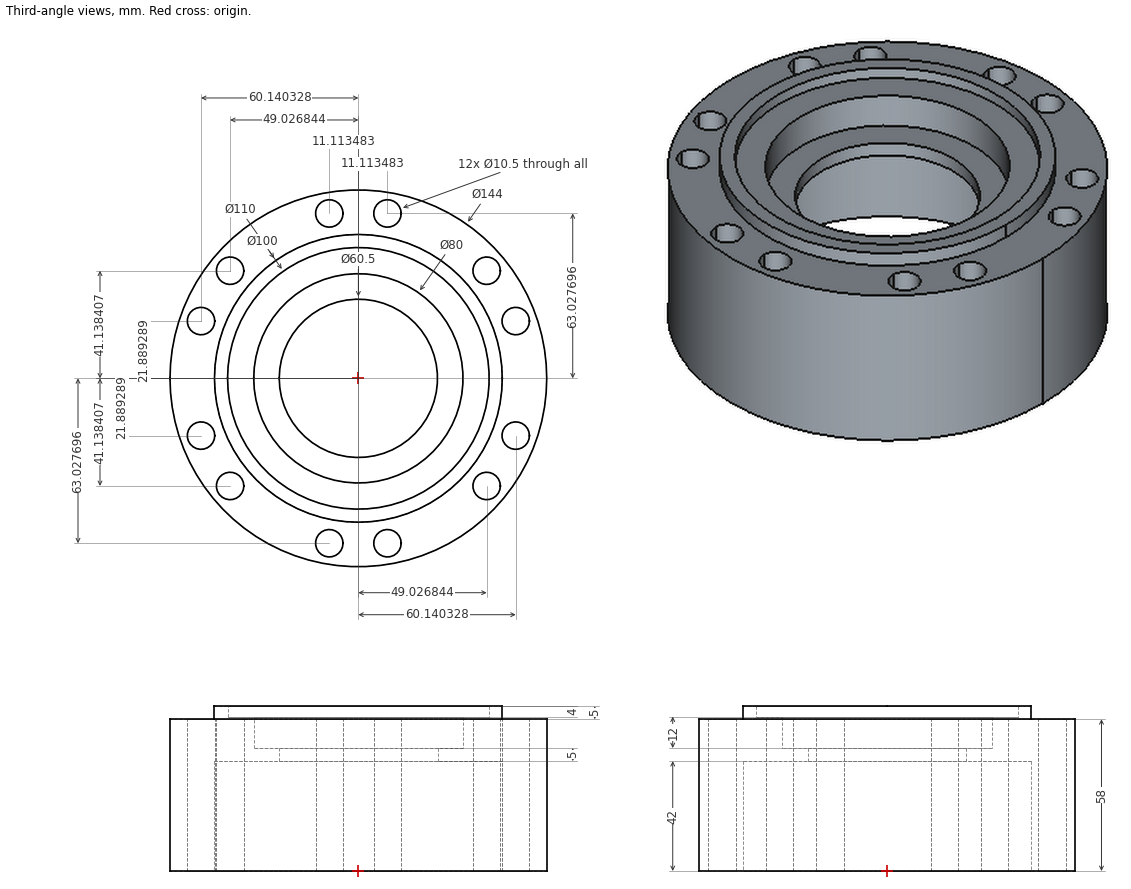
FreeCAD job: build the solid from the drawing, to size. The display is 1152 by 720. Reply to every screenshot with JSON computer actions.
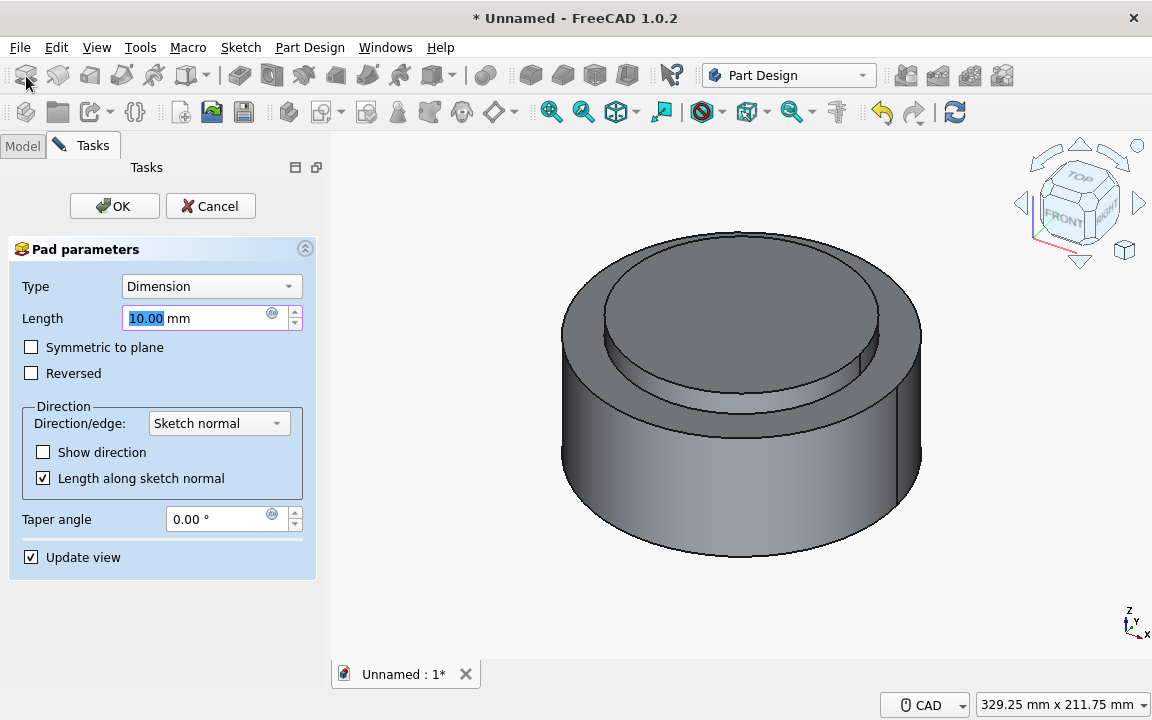
{"action": "type", "text": "5"}
{"action": "key", "text": "Tab"}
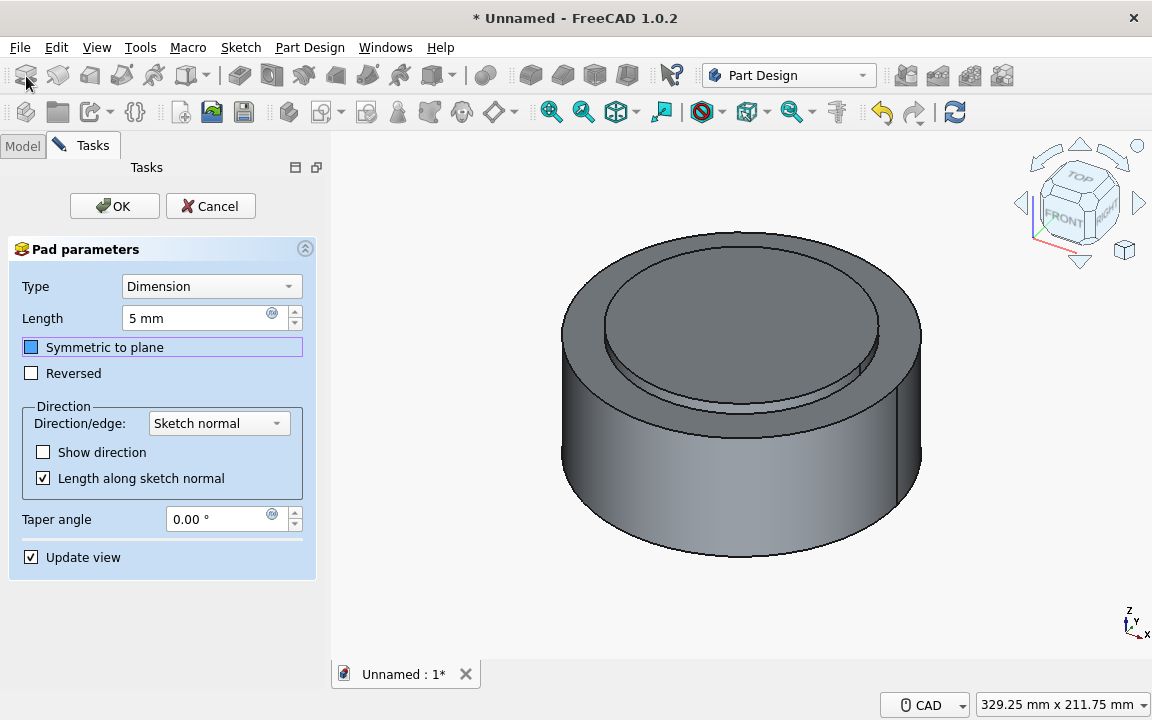
{"action": "left_click", "coordinate": [115, 206]}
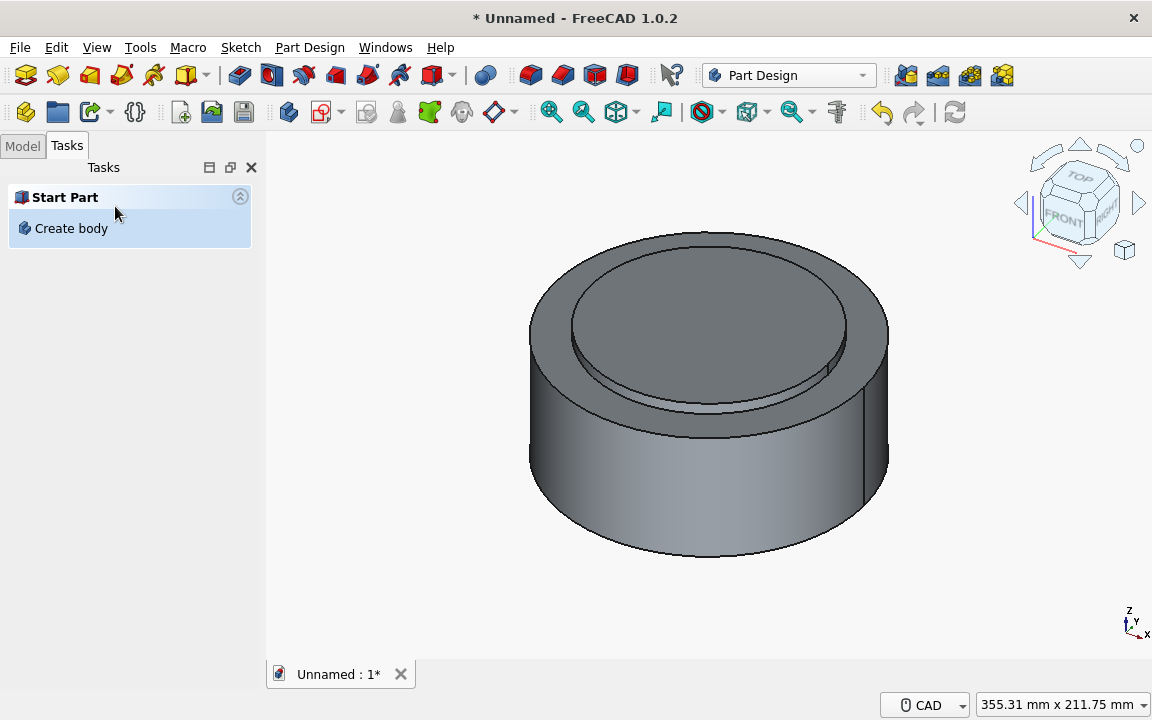
{"action": "key", "text": "5"}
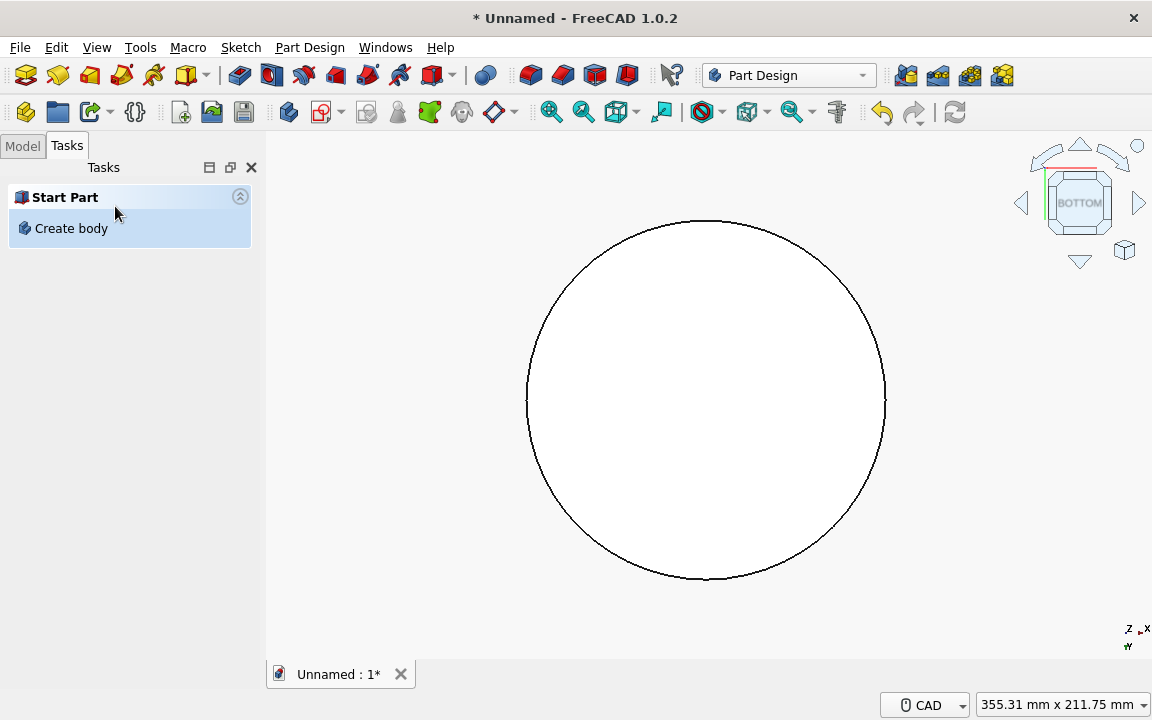
{"action": "left_click", "coordinate": [706, 399]}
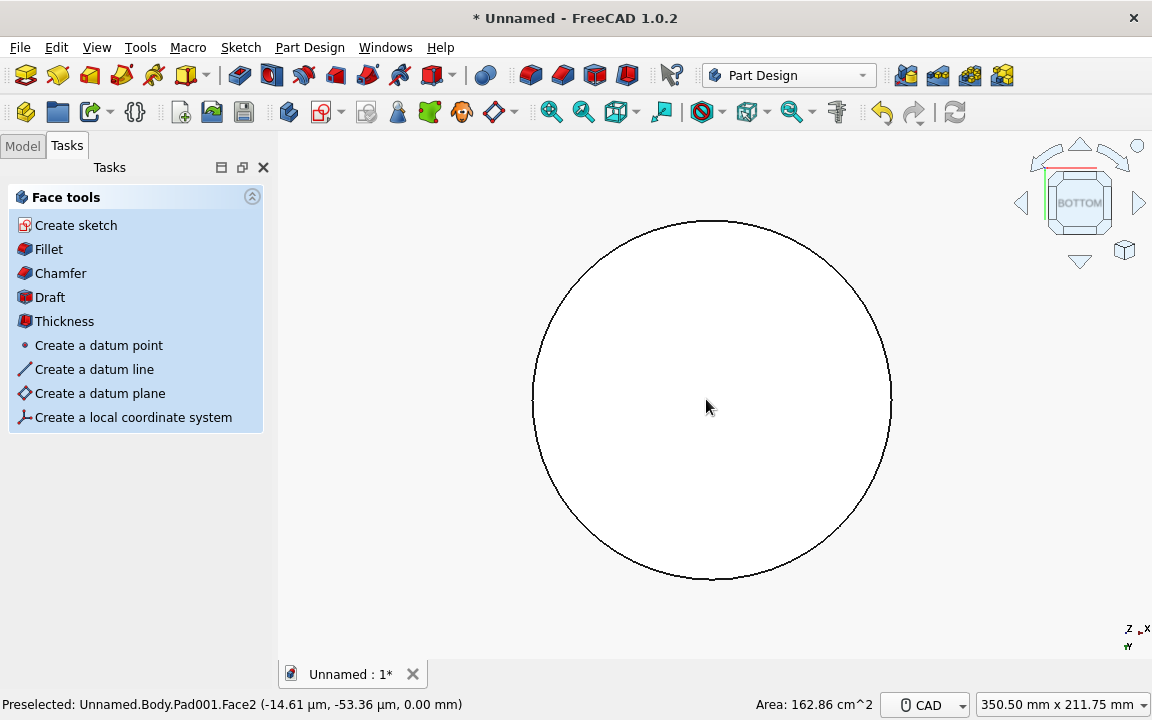
{"action": "left_click", "coordinate": [322, 112]}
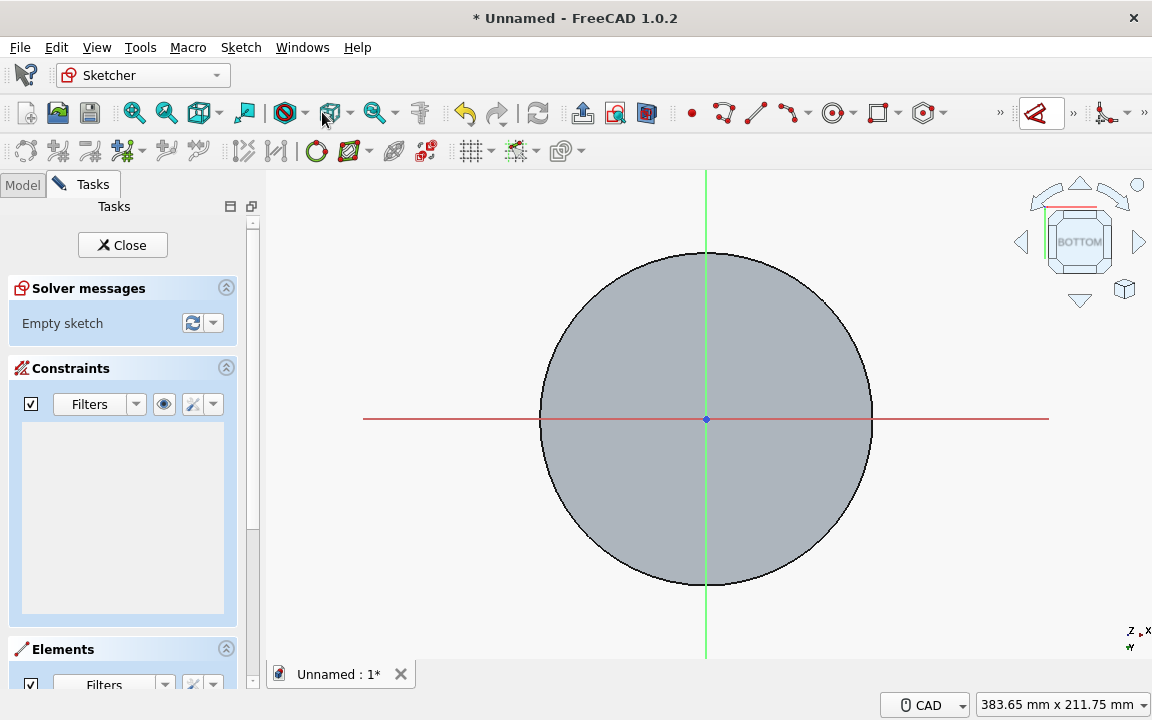
{"action": "left_click", "coordinate": [834, 114]}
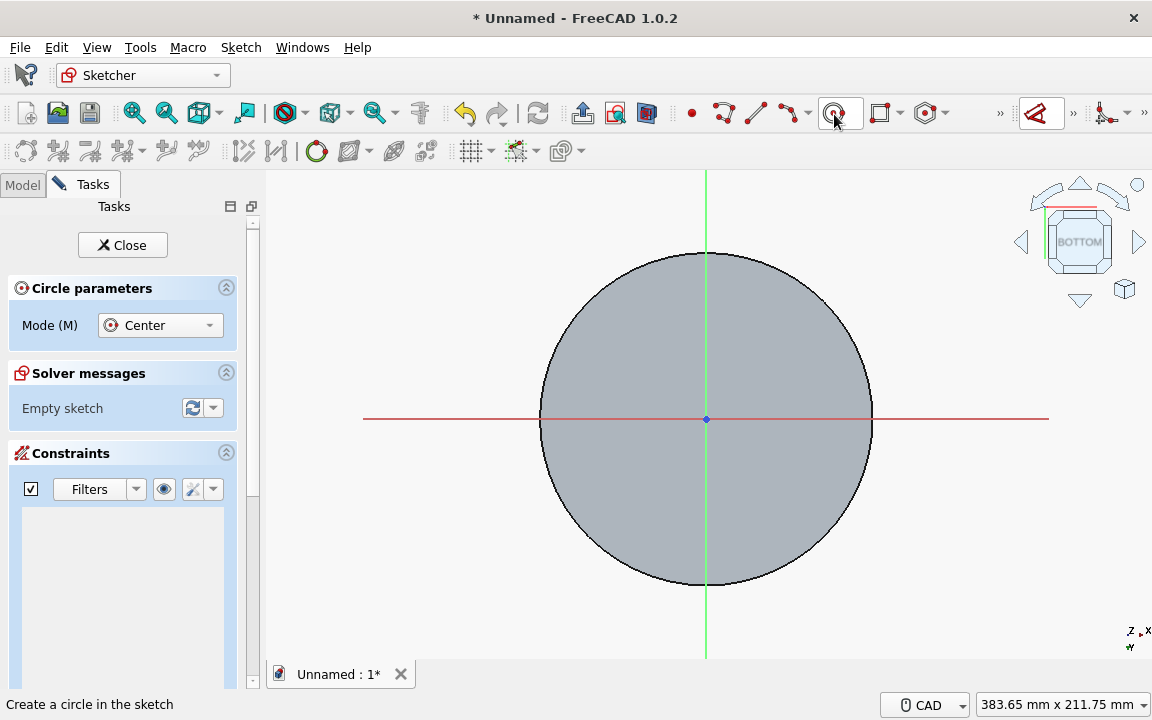
{"action": "scroll", "coordinate": [732, 565], "scroll_direction": "up", "scroll_amount": 4}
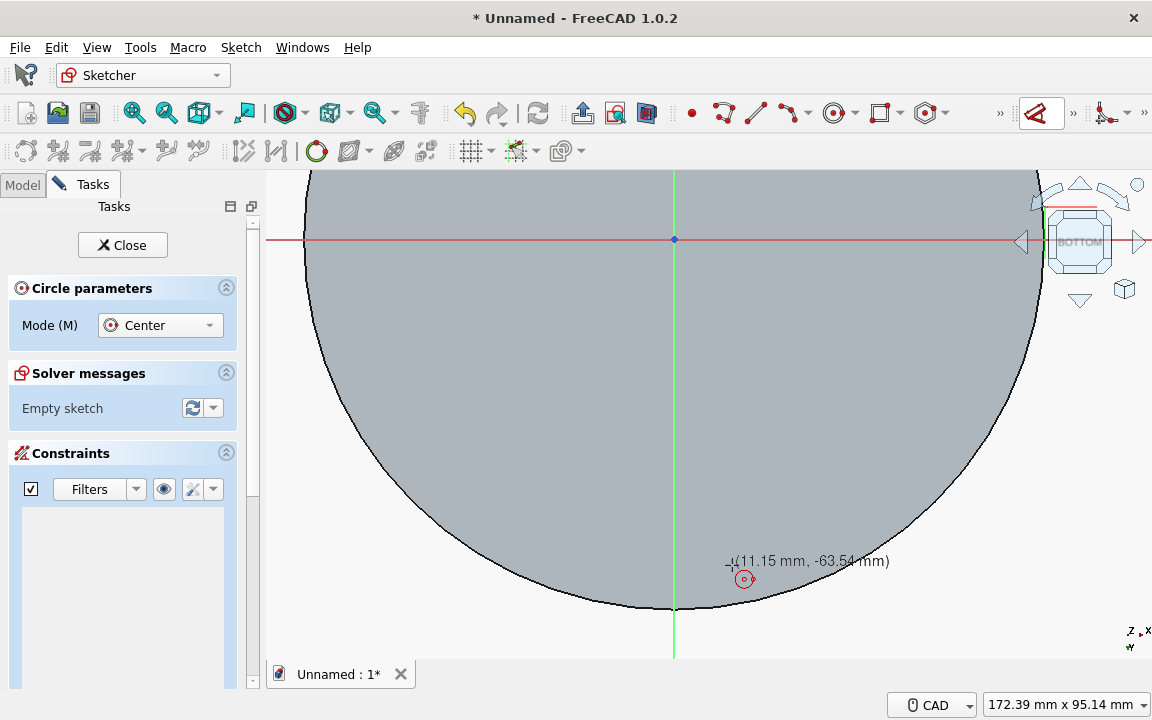
{"action": "left_click", "coordinate": [731, 564]}
{"action": "left_click", "coordinate": [750, 545]}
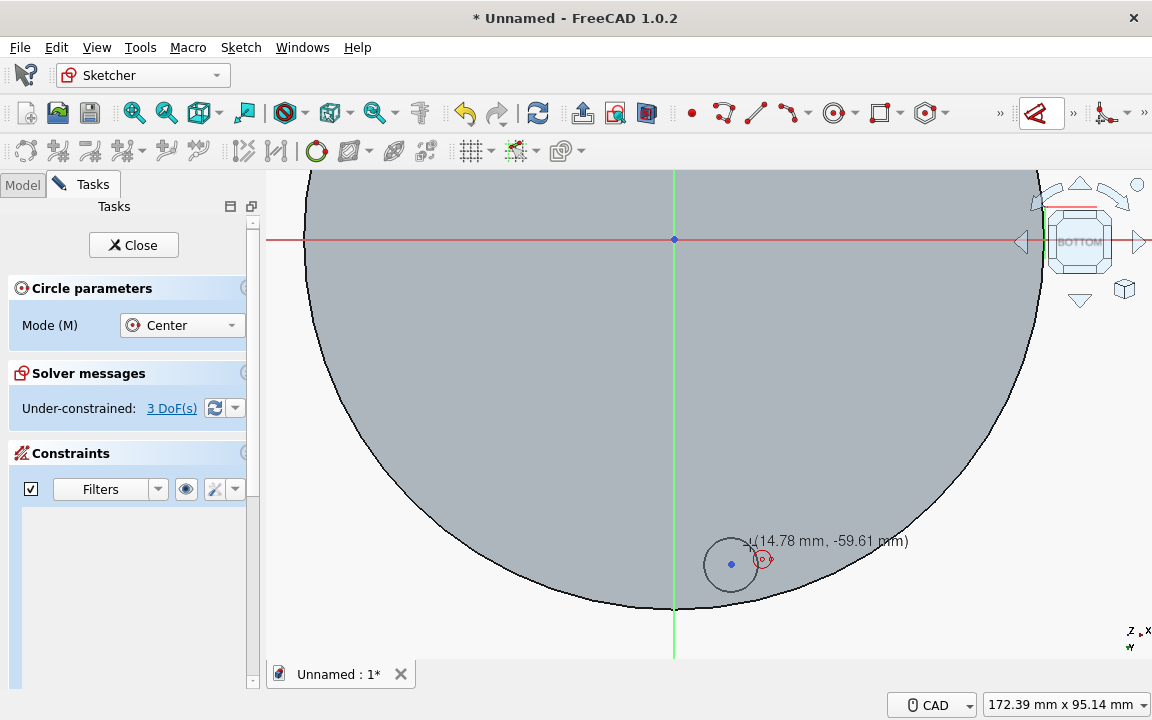
{"action": "left_click", "coordinate": [617, 564]}
{"action": "left_click", "coordinate": [636, 545]}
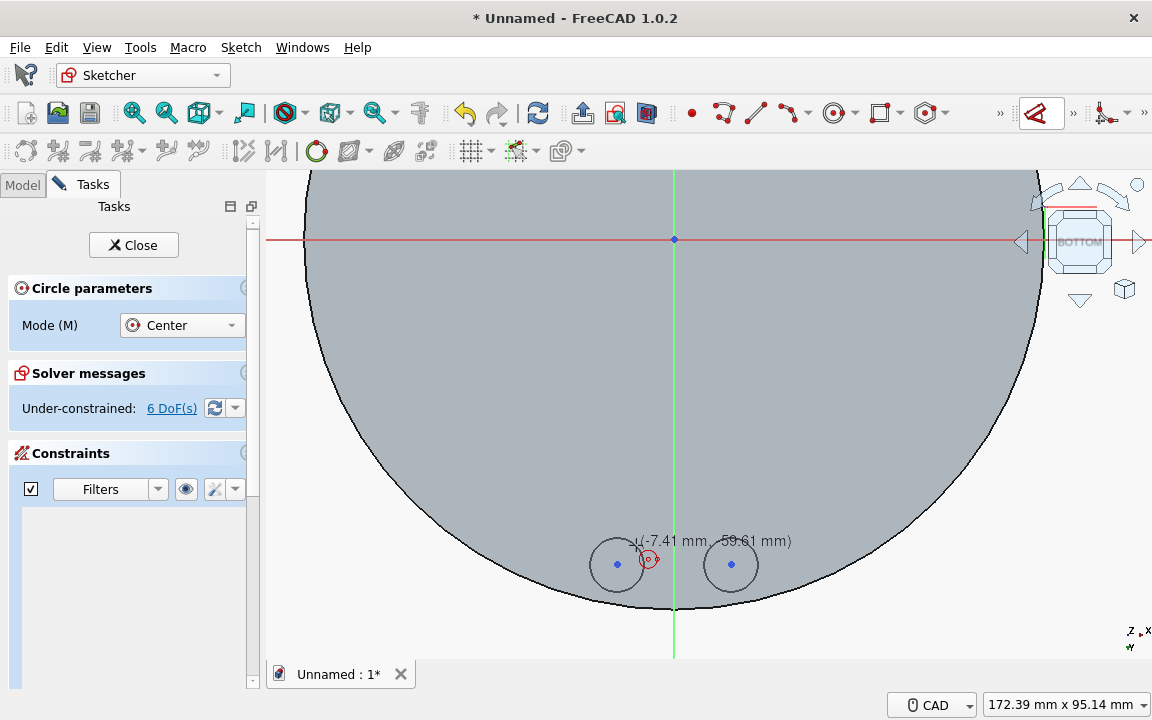
{"action": "left_click", "coordinate": [422, 451]}
{"action": "left_click", "coordinate": [441, 432]}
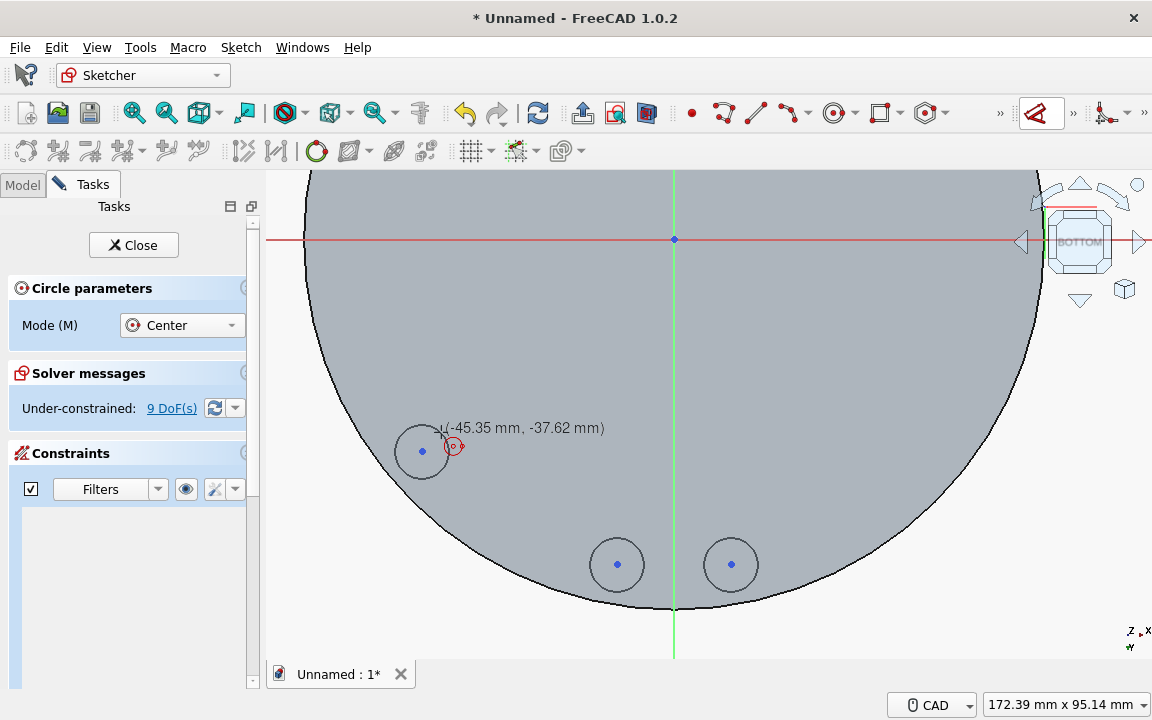
{"action": "left_click", "coordinate": [365, 352]}
{"action": "left_click", "coordinate": [384, 333]}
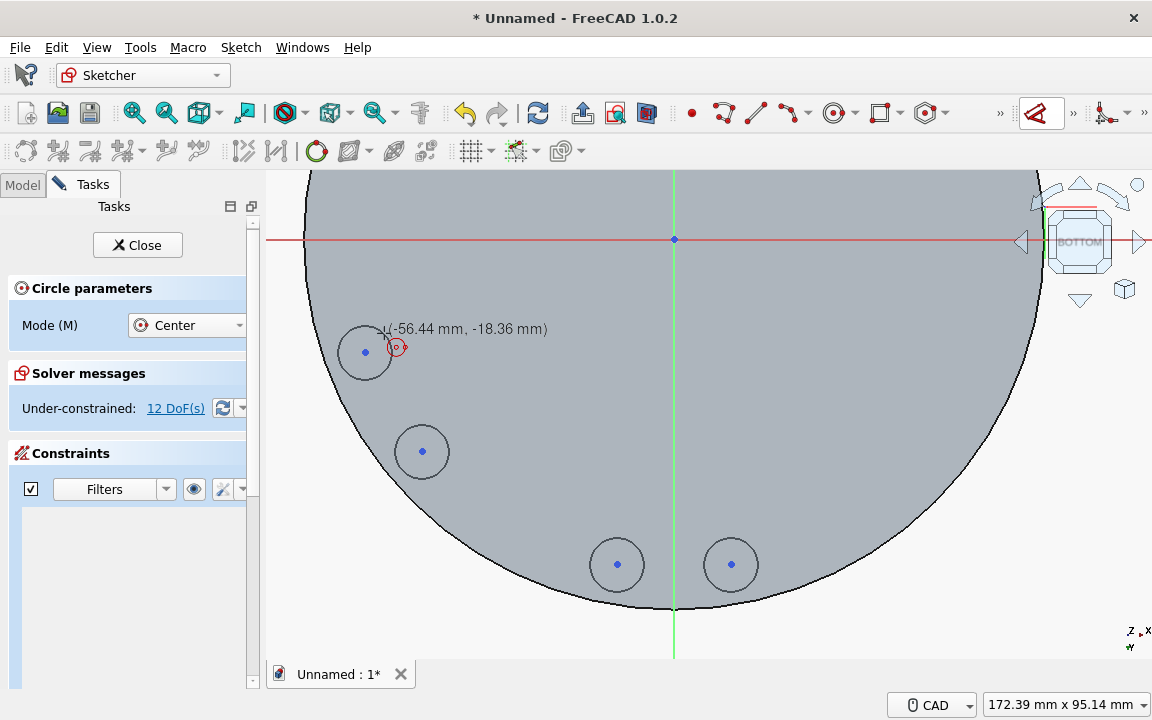
{"action": "scroll", "coordinate": [613, 557], "scroll_direction": "down", "scroll_amount": 4}